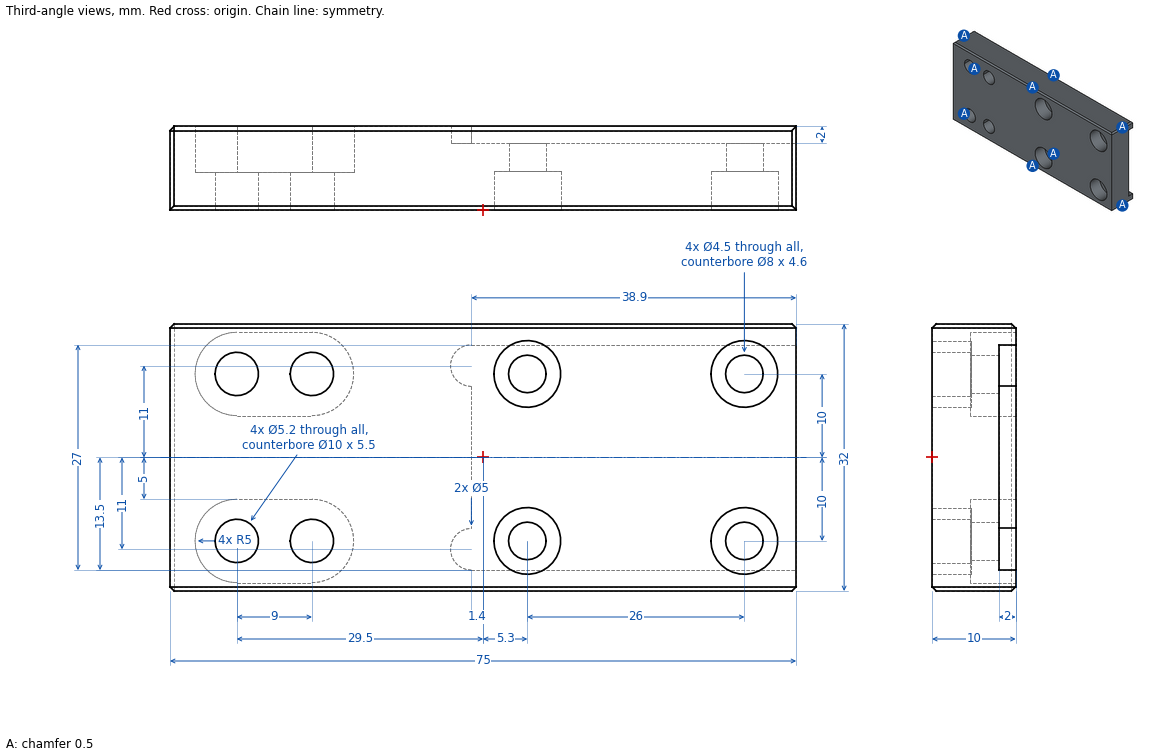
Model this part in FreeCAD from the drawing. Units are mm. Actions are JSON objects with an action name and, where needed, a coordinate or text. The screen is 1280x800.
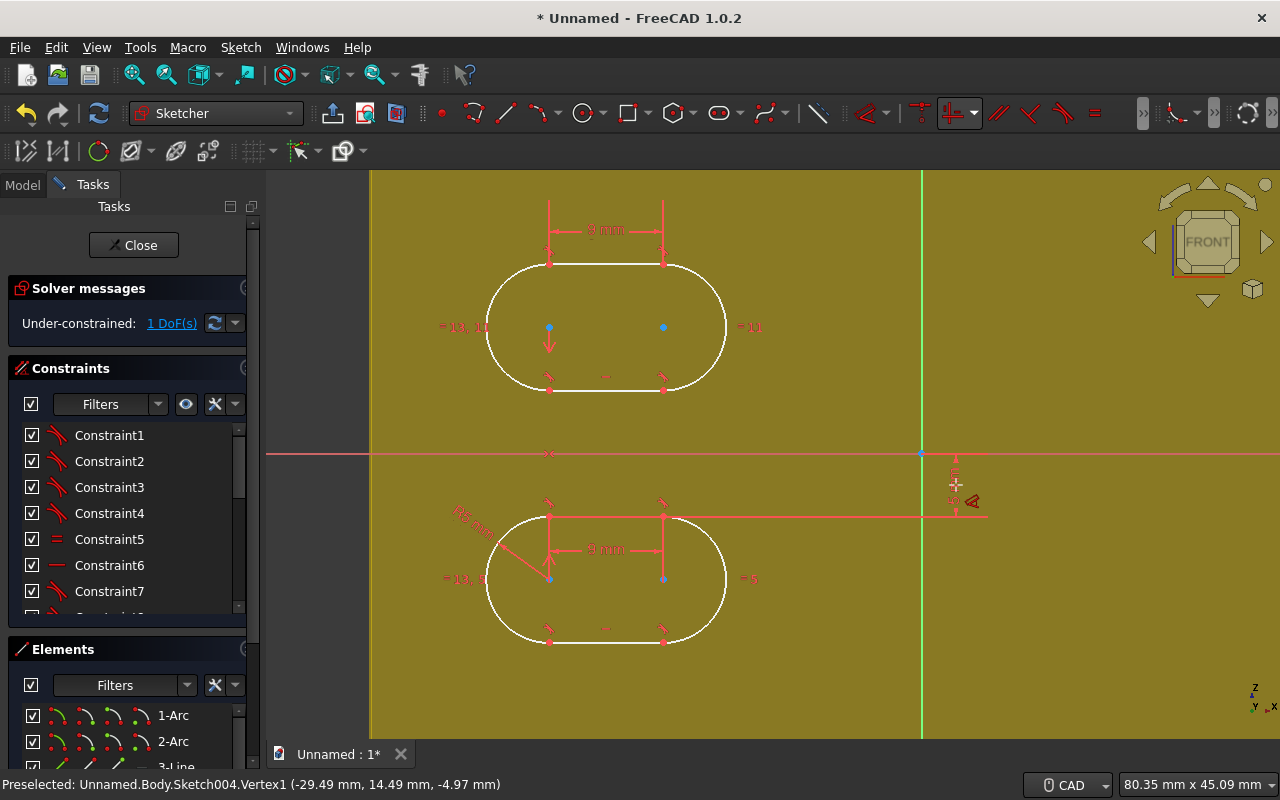
{"action": "left_click", "coordinate": [549, 517]}
{"action": "left_click", "coordinate": [735, 551]}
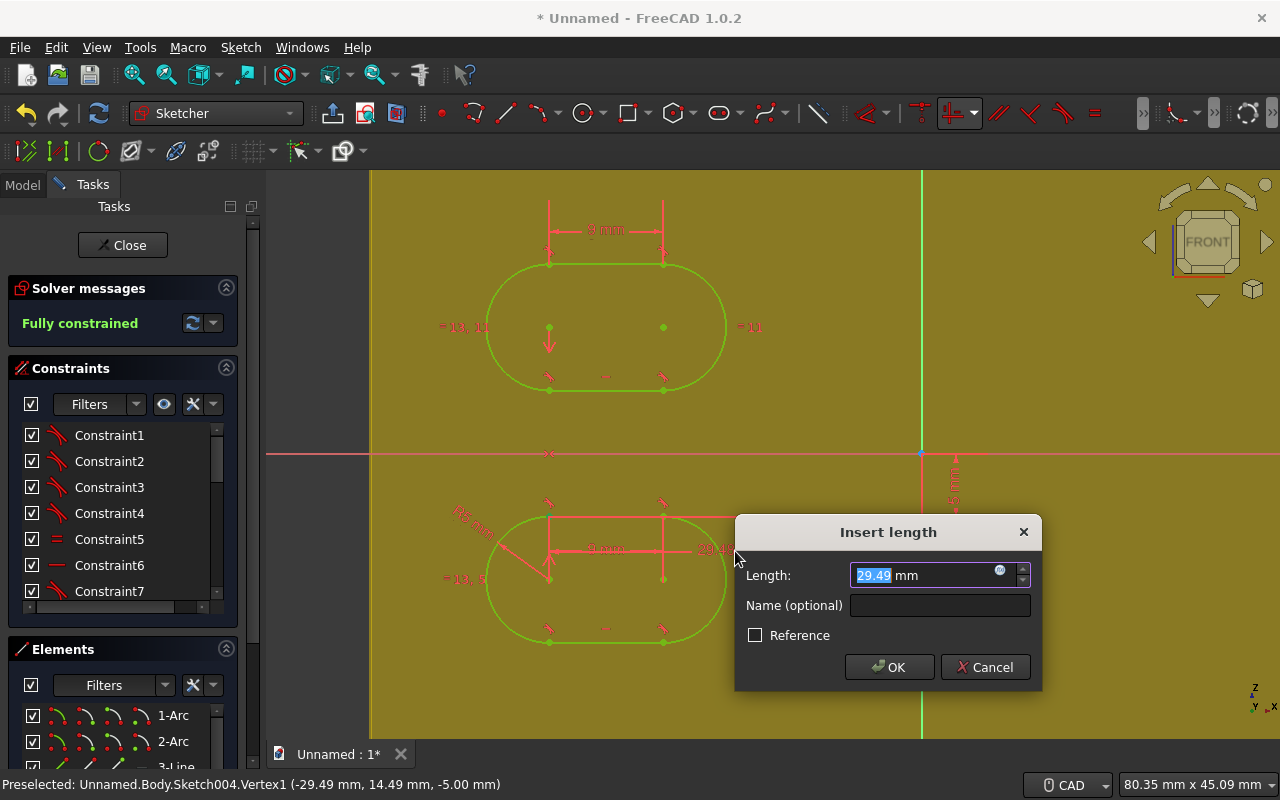
{"action": "type", "text": "29.5"}
{"action": "key", "text": "Return"}
{"action": "key", "text": "Escape"}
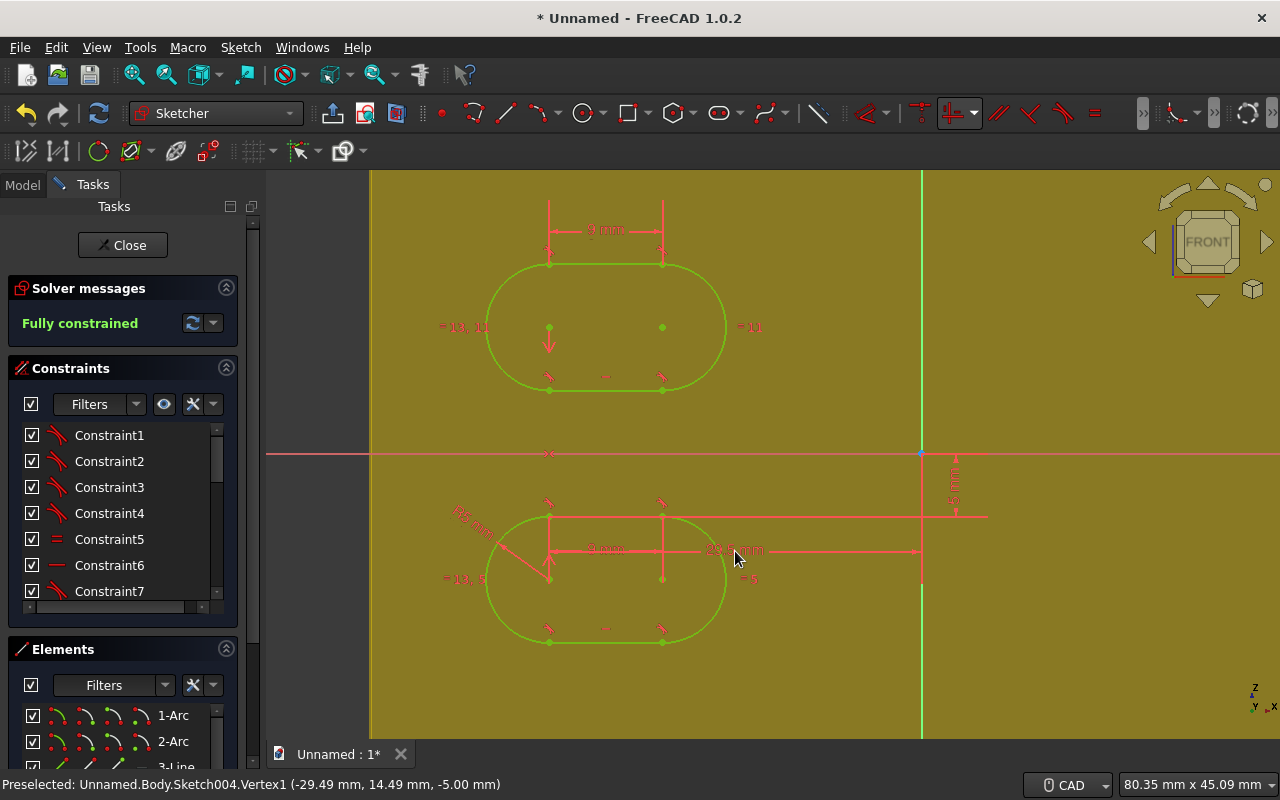
{"action": "left_click", "coordinate": [123, 245]}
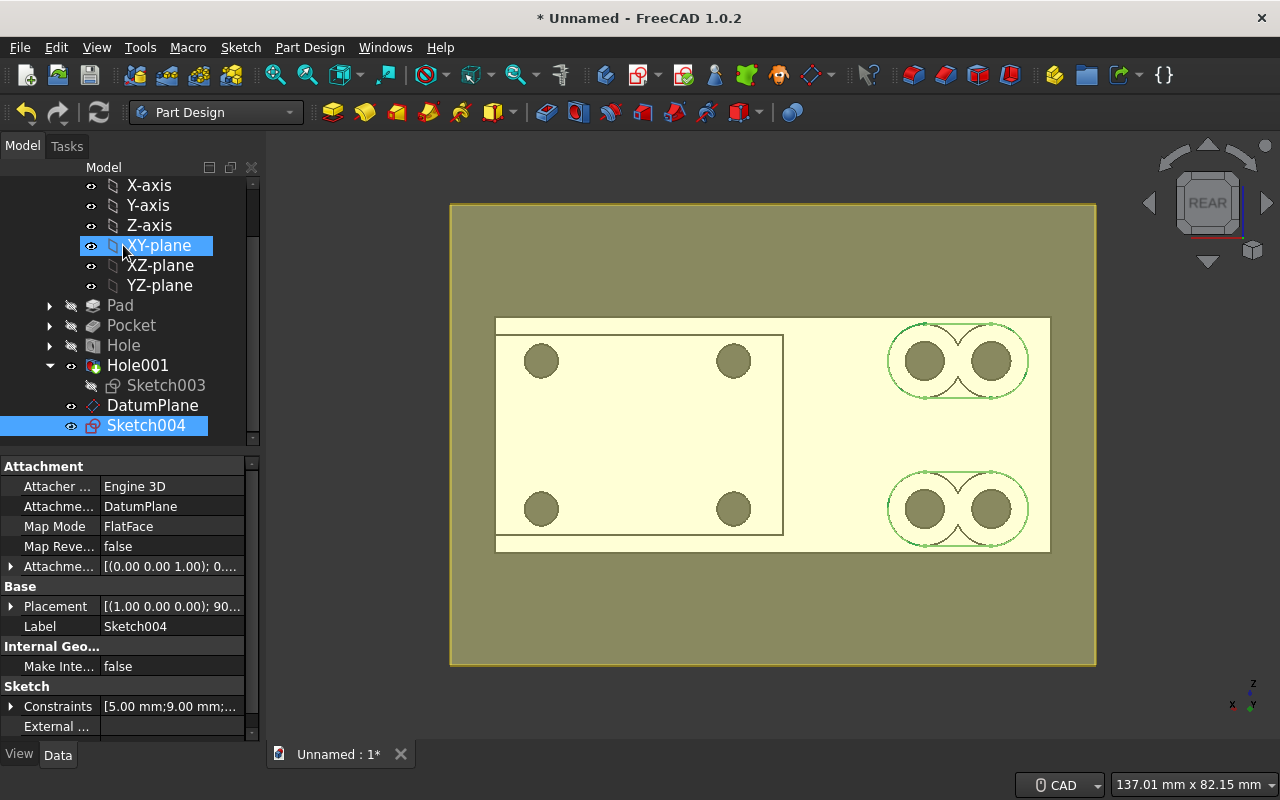
{"action": "left_click", "coordinate": [548, 112]}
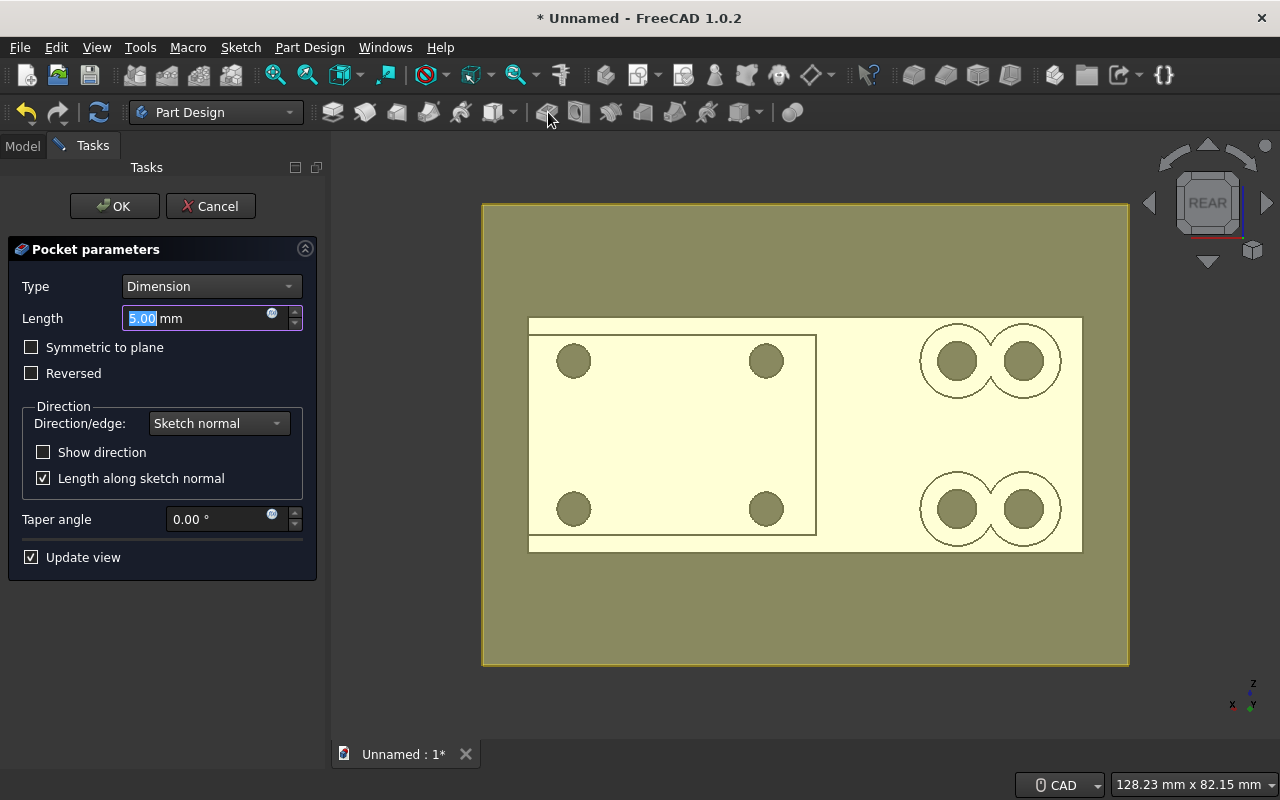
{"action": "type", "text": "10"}
{"action": "key", "text": "Tab"}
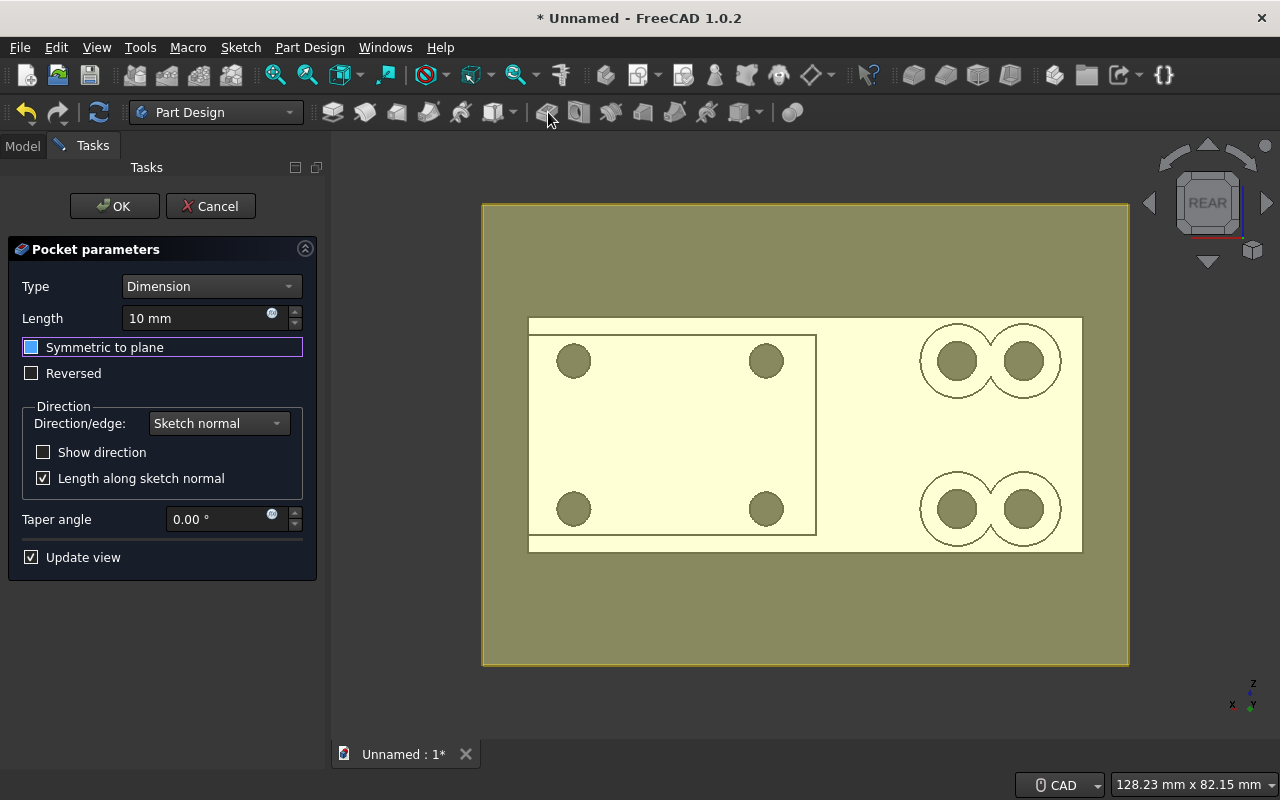
{"action": "left_click", "coordinate": [30, 373]}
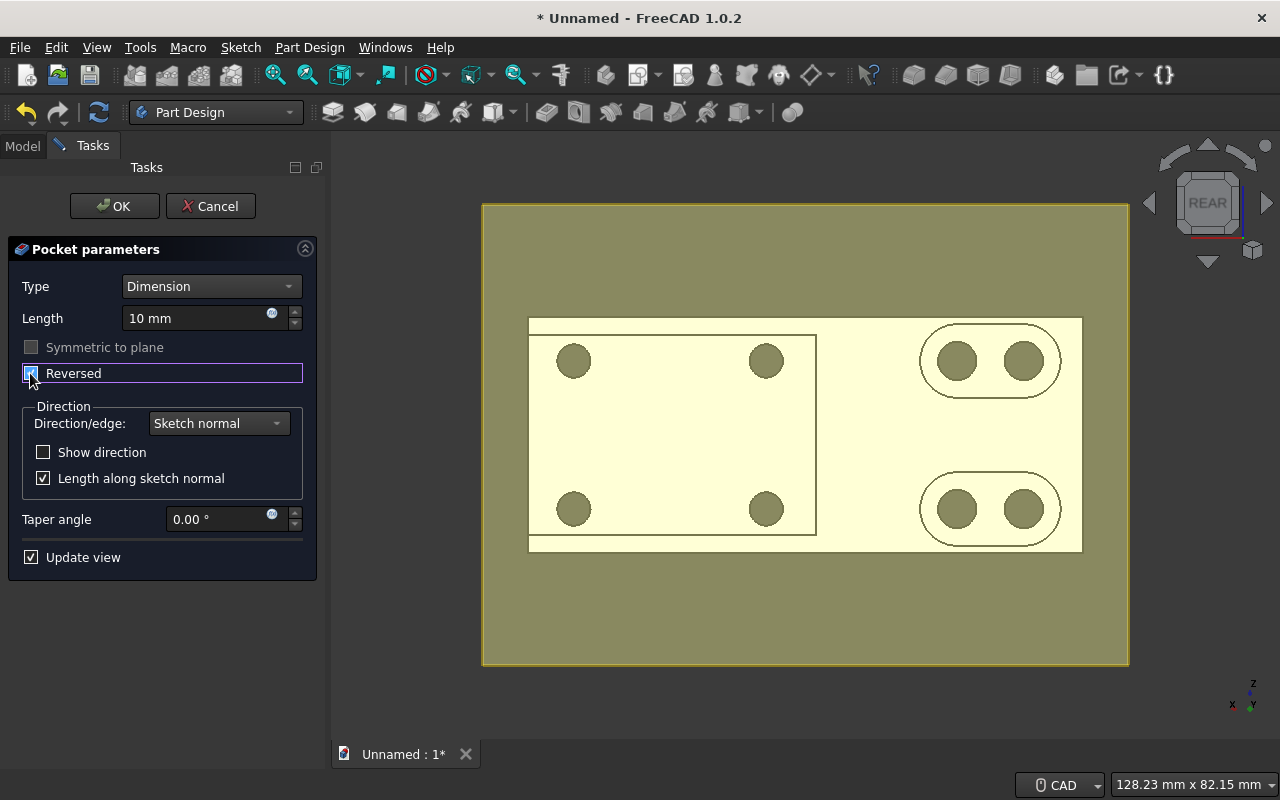
{"action": "left_click", "coordinate": [115, 206]}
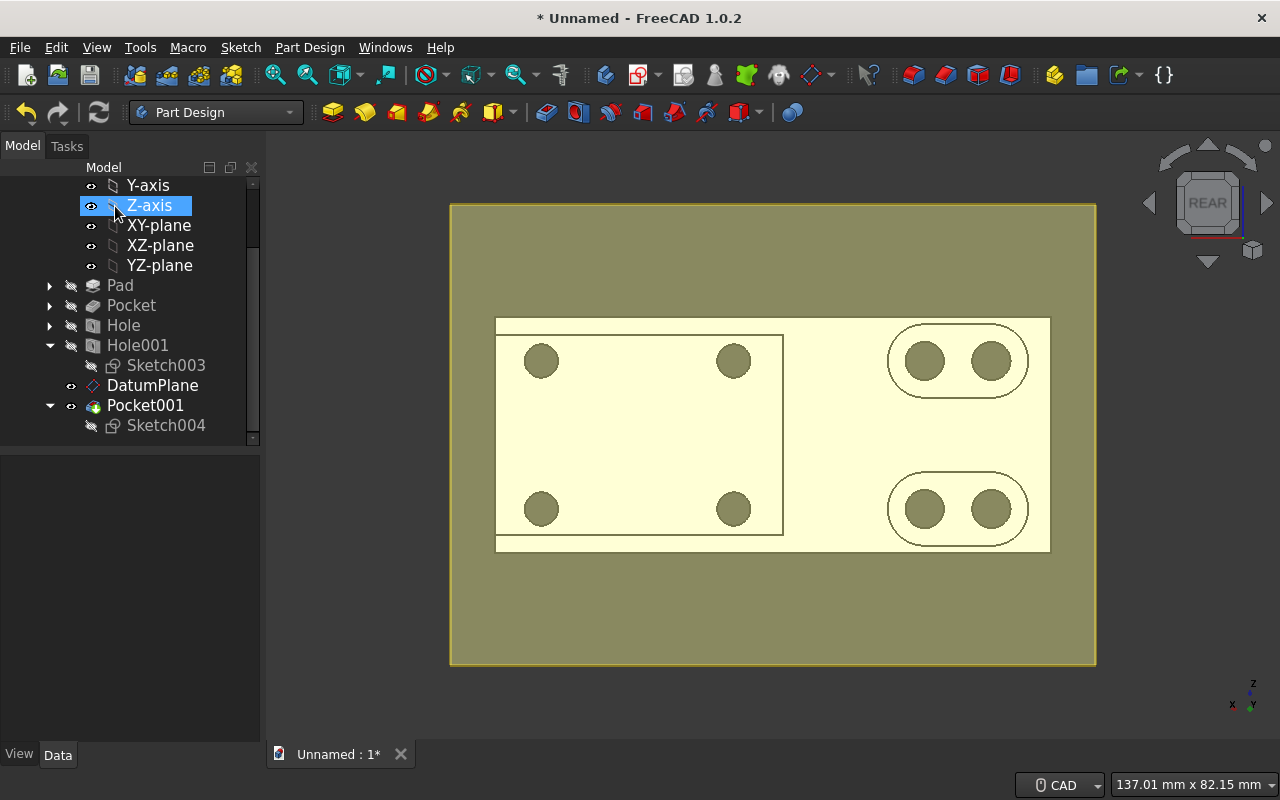
{"action": "left_click", "coordinate": [116, 386]}
{"action": "key", "text": "space"}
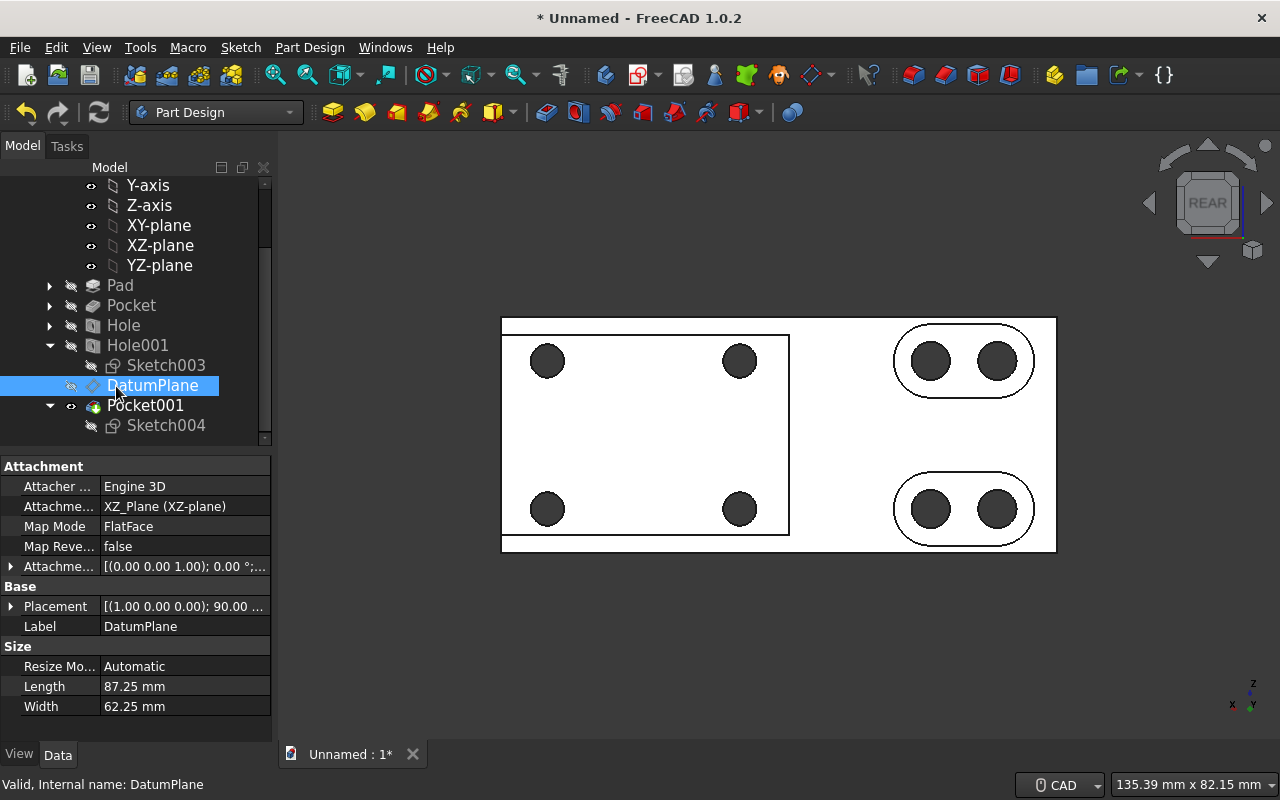
{"action": "left_click", "coordinate": [858, 434]}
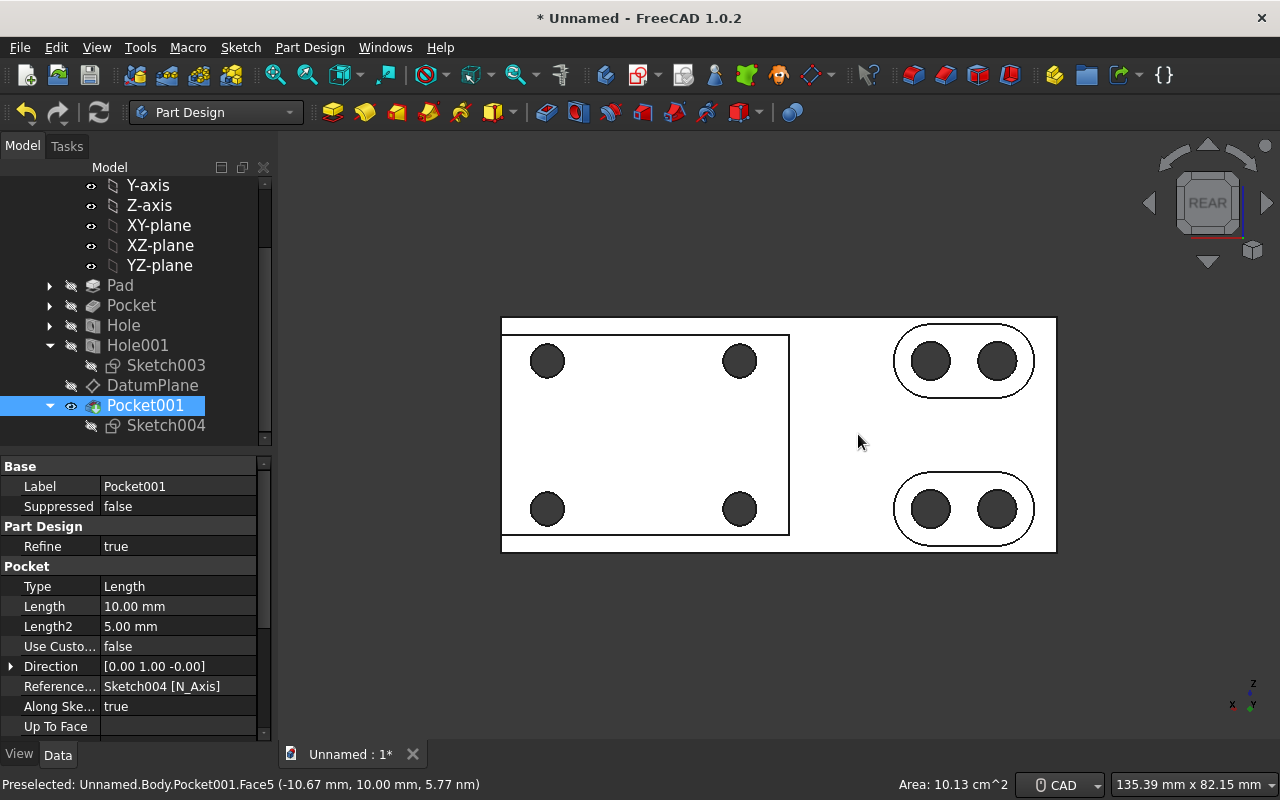
{"action": "left_click", "coordinate": [638, 76]}